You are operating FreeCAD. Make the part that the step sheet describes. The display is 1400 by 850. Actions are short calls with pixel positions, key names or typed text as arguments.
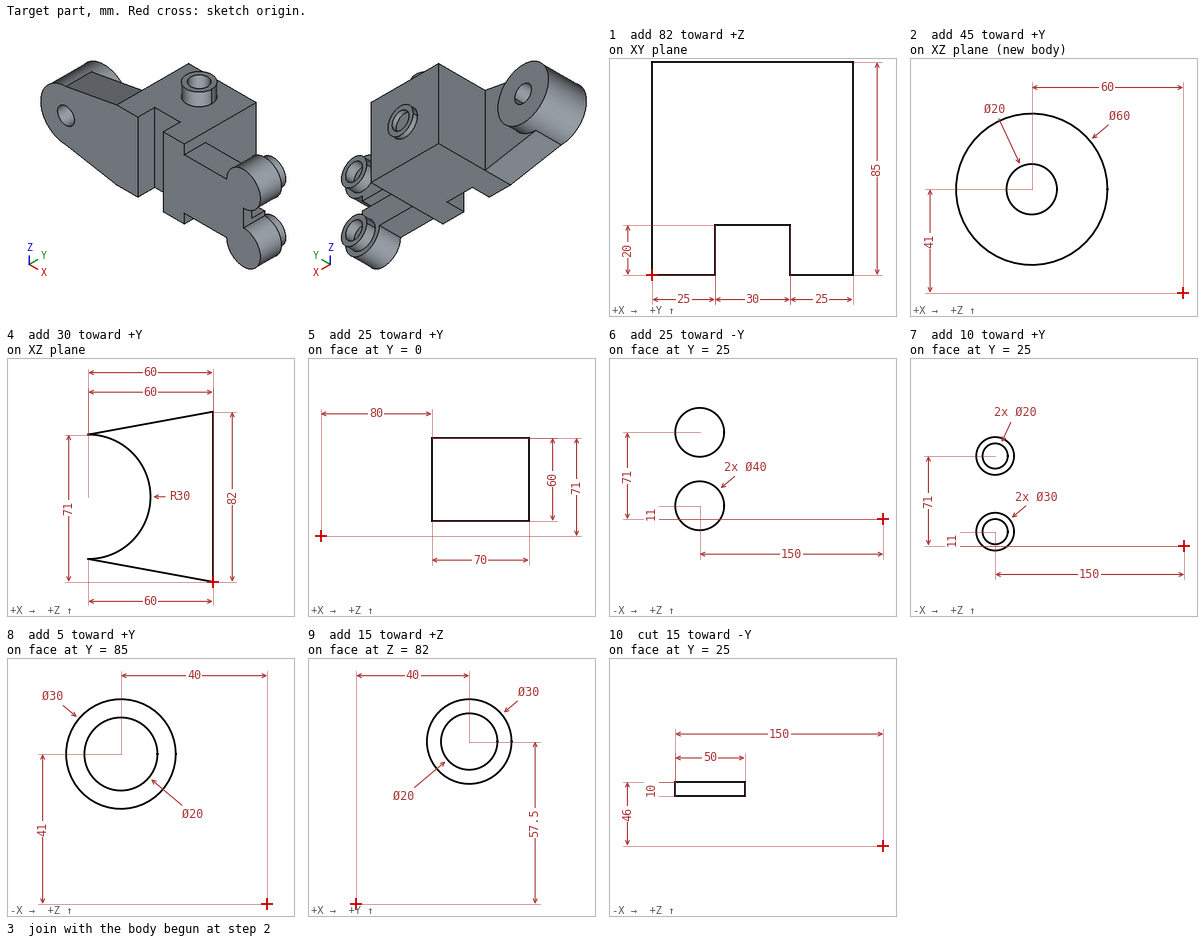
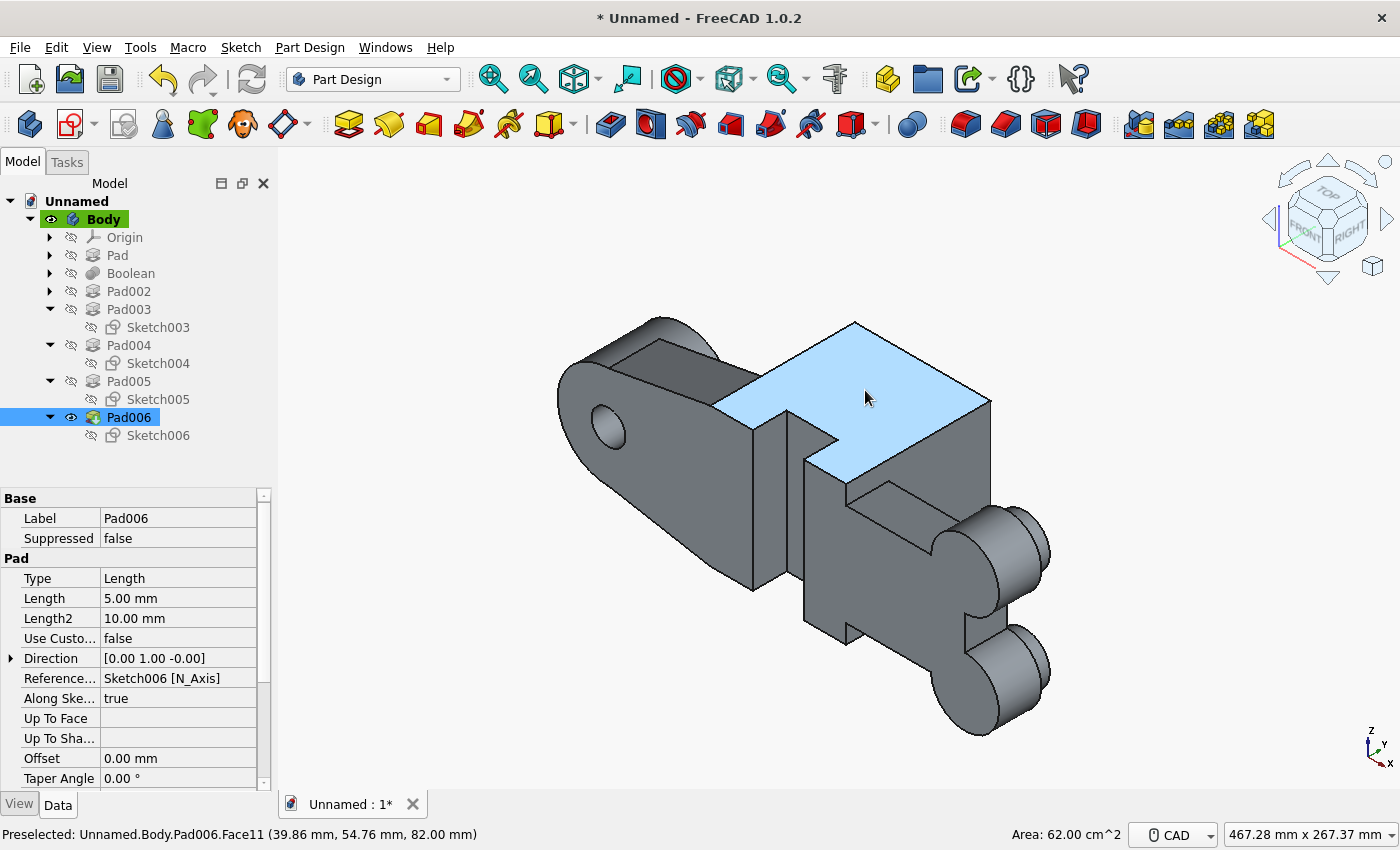
click(70, 124)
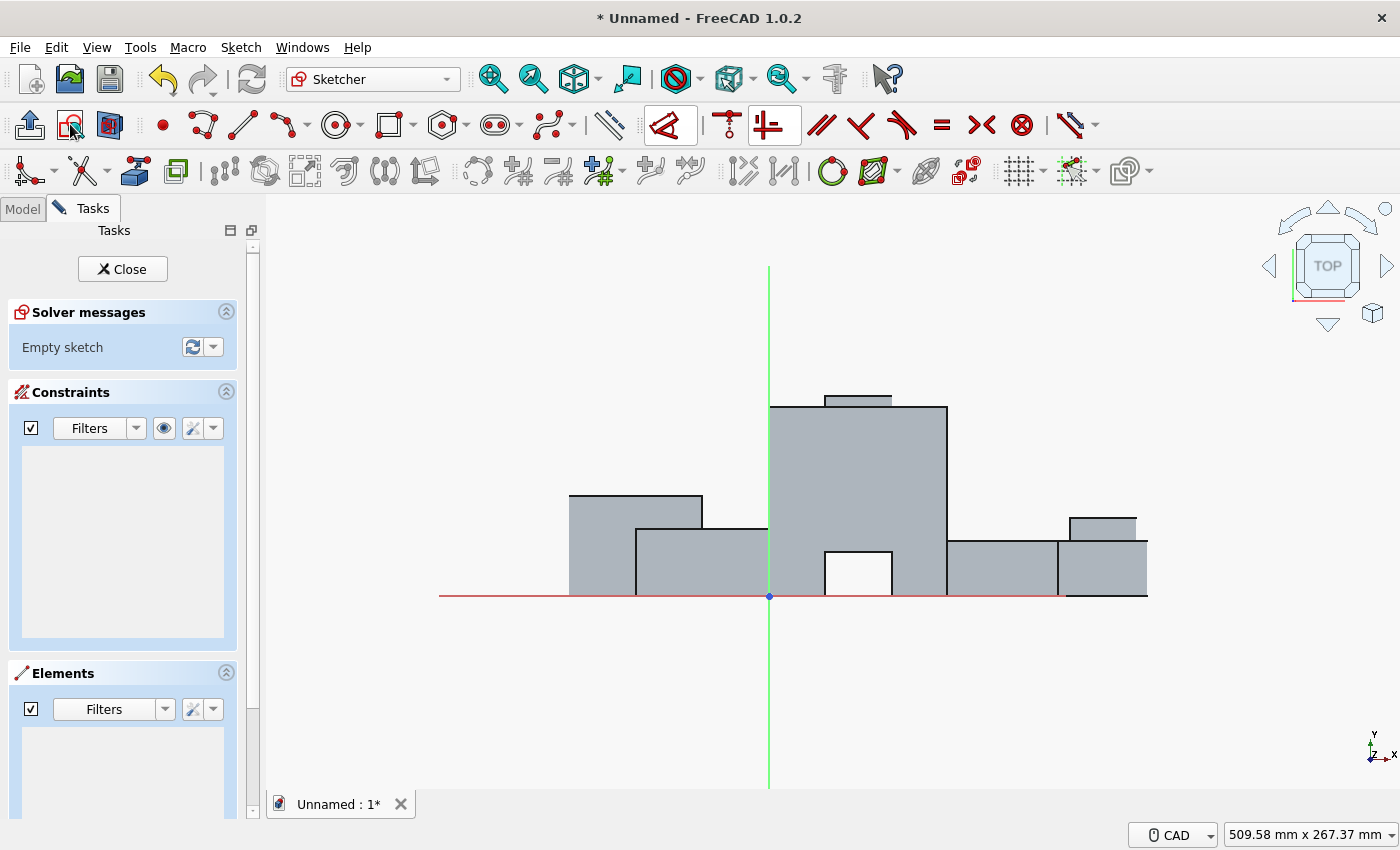
click(110, 126)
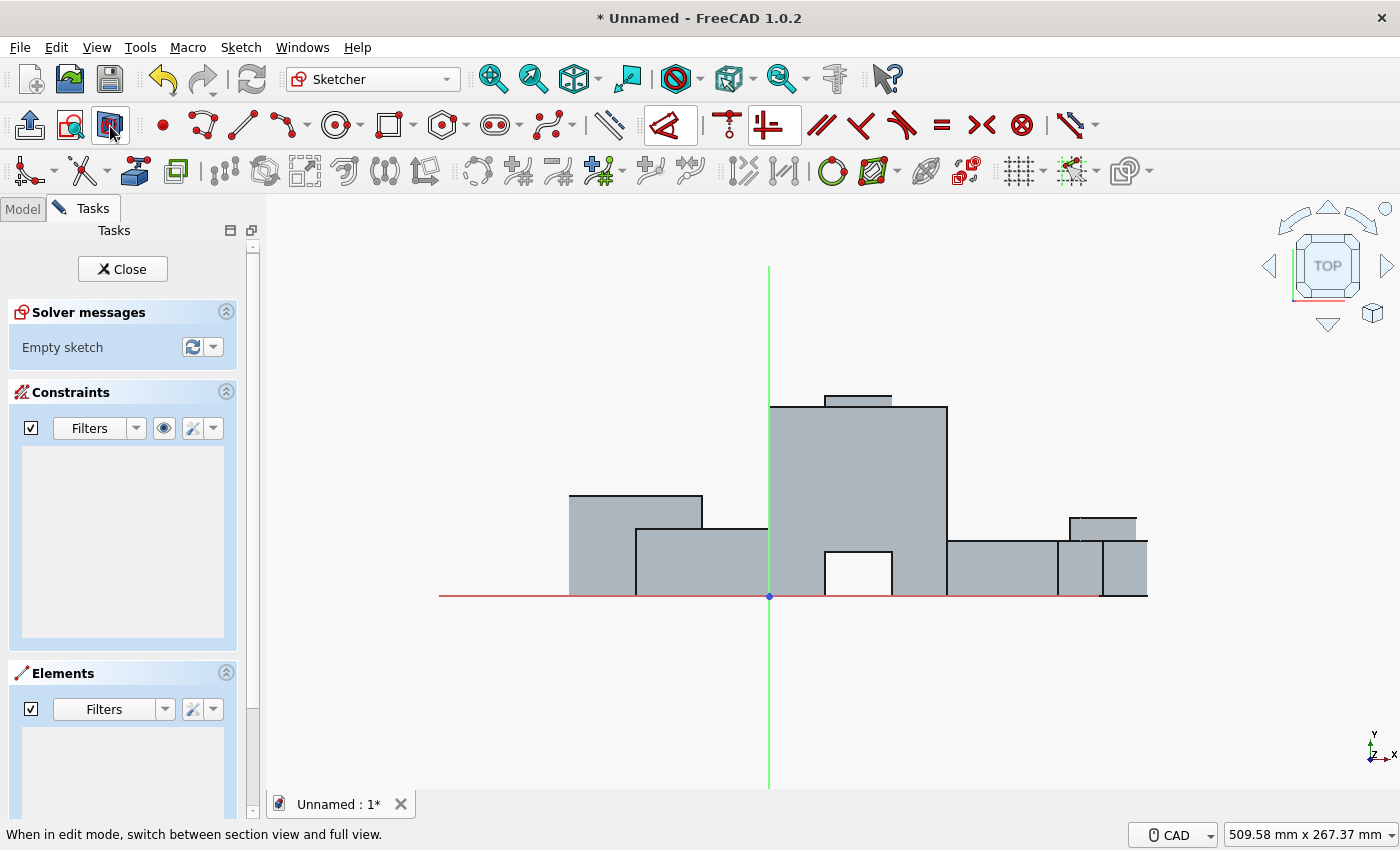
scroll(884, 535, up, 4)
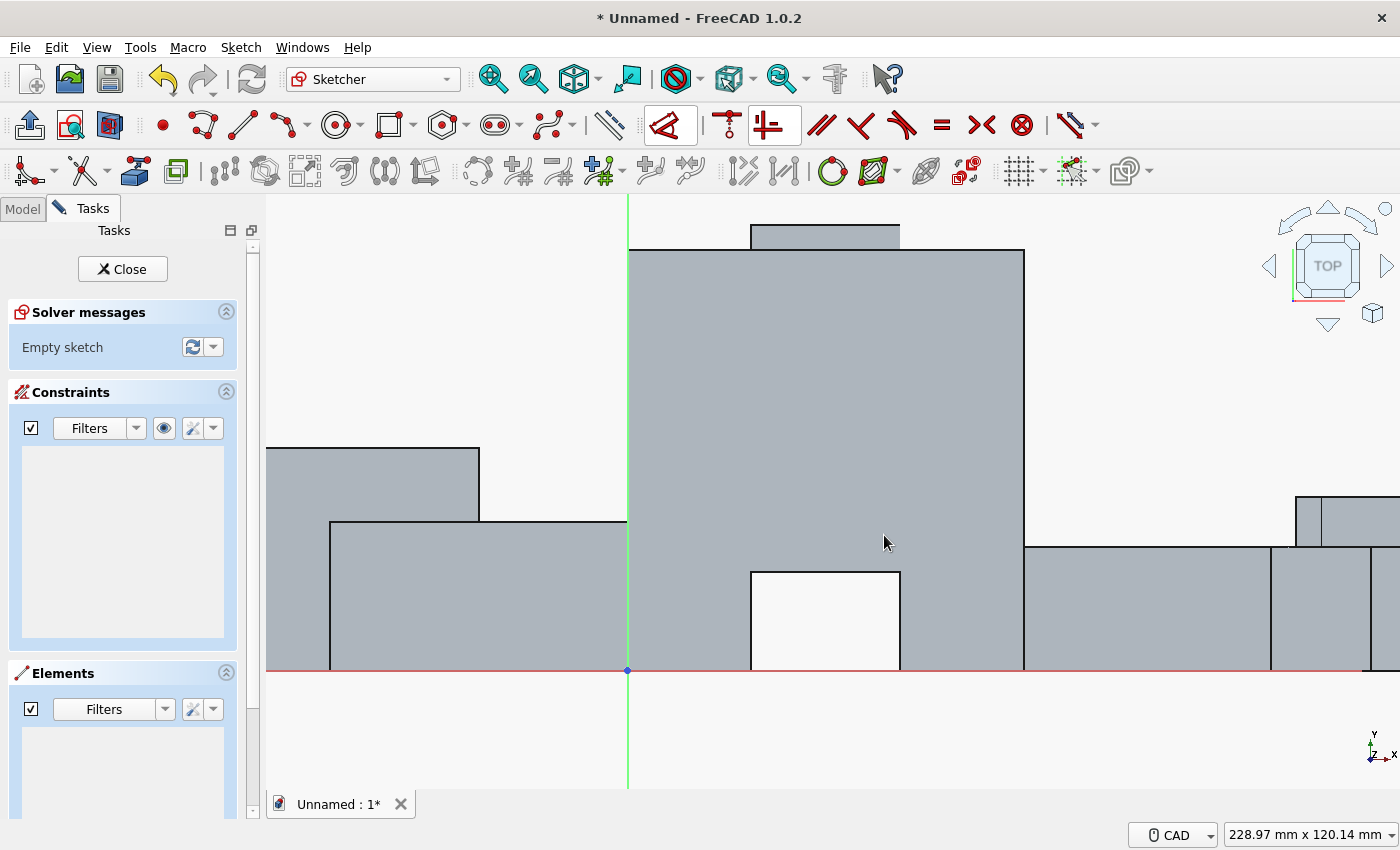
click(336, 126)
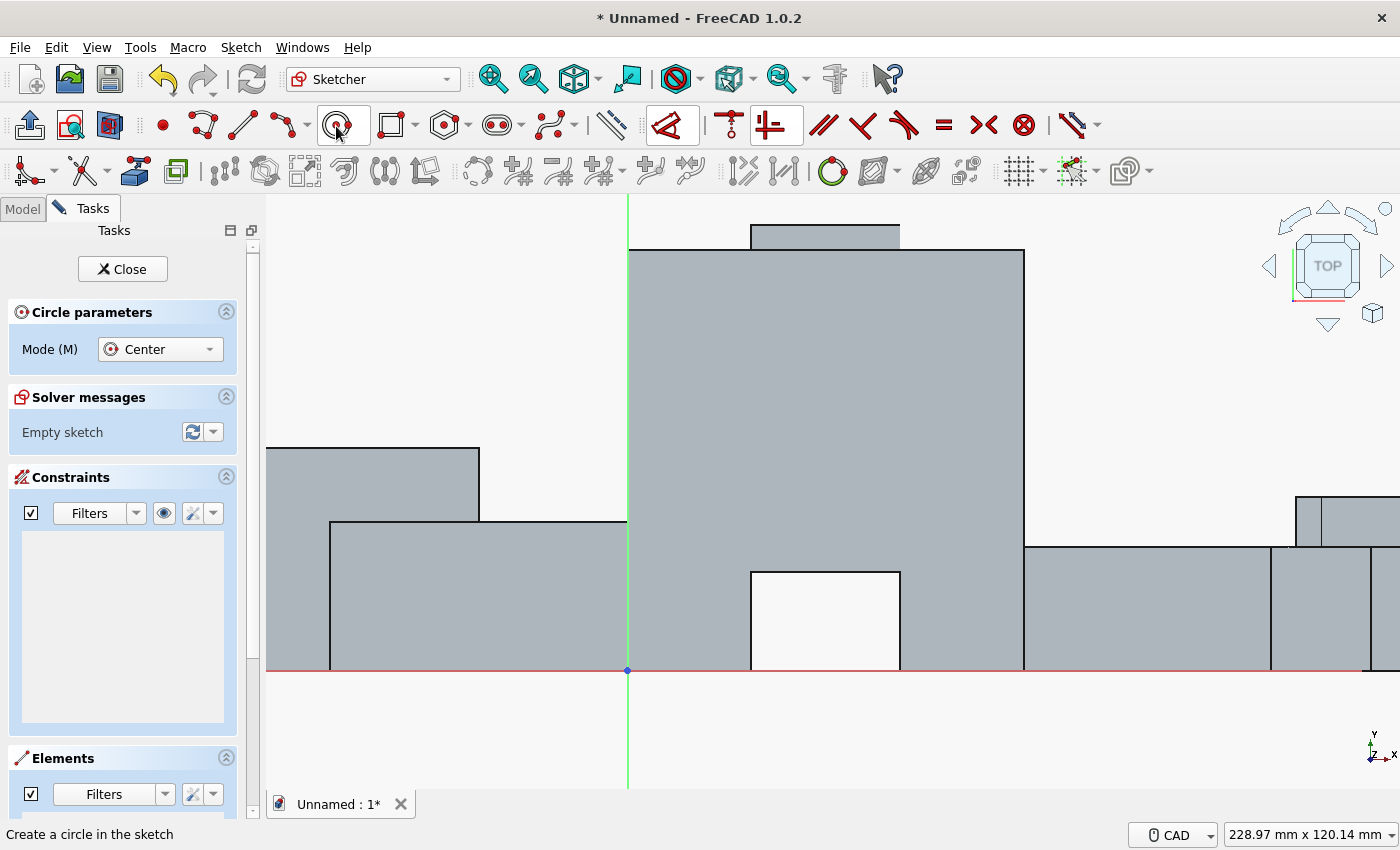
click(826, 386)
click(878, 333)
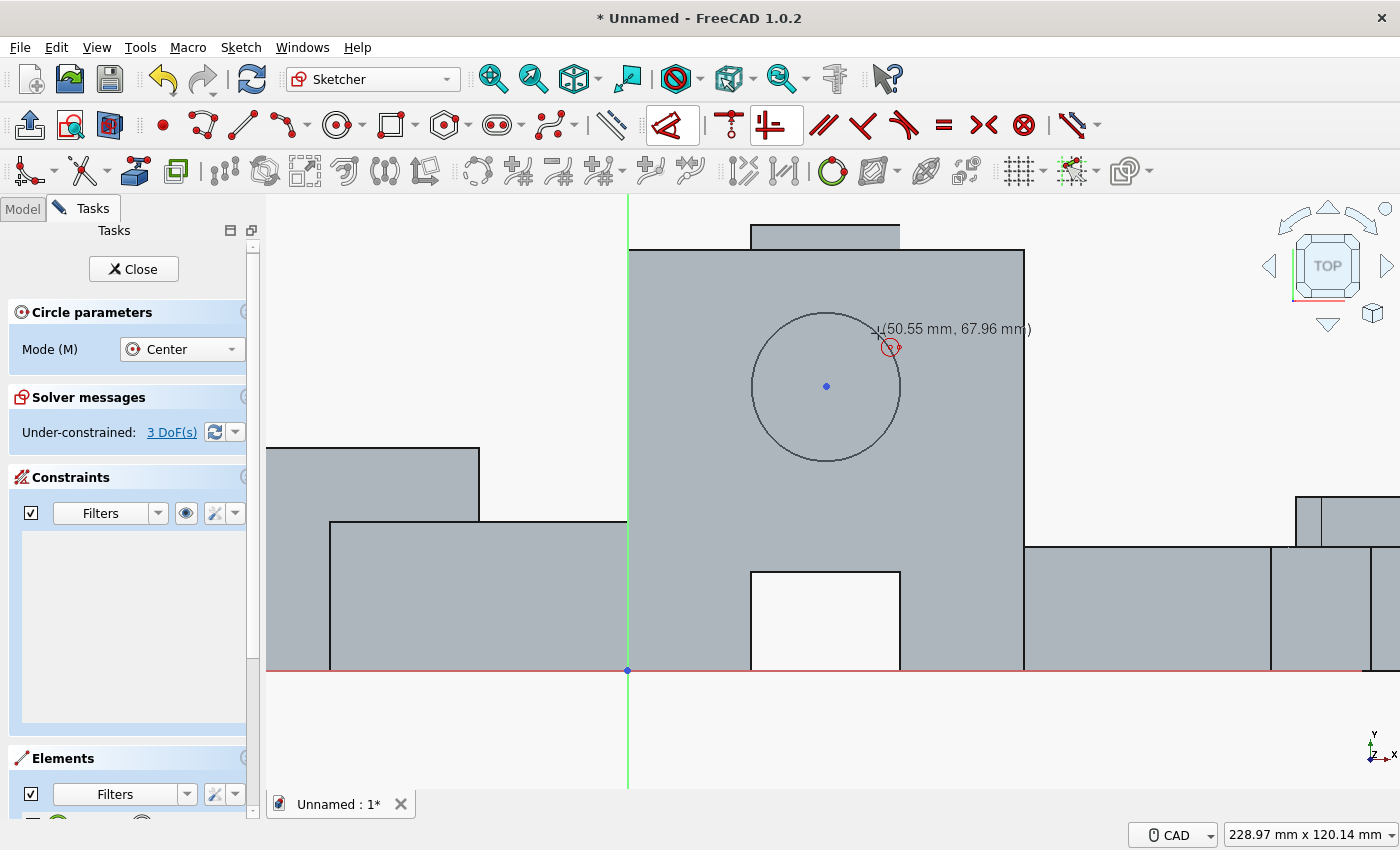
click(826, 387)
click(861, 351)
key(Escape)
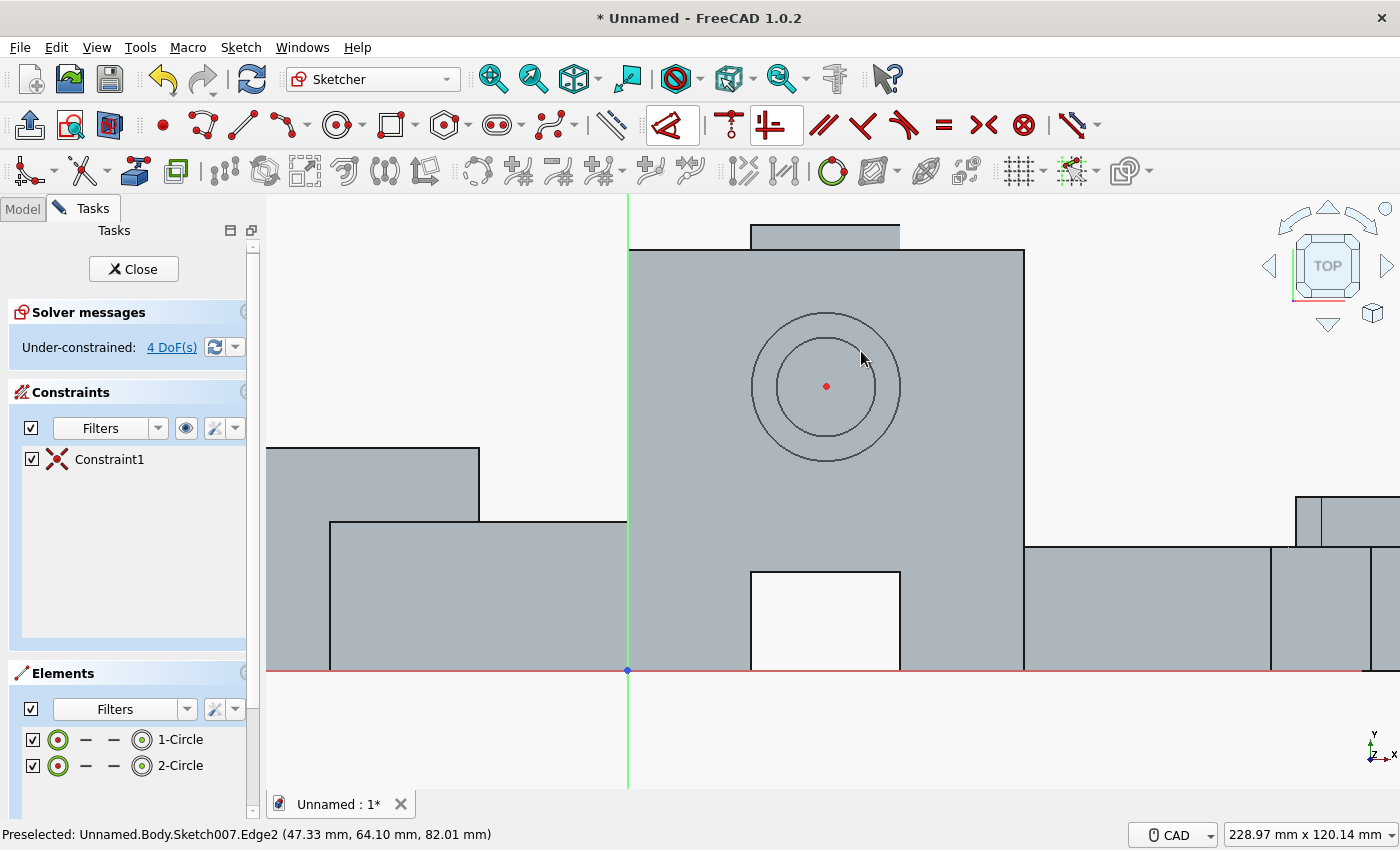
click(878, 334)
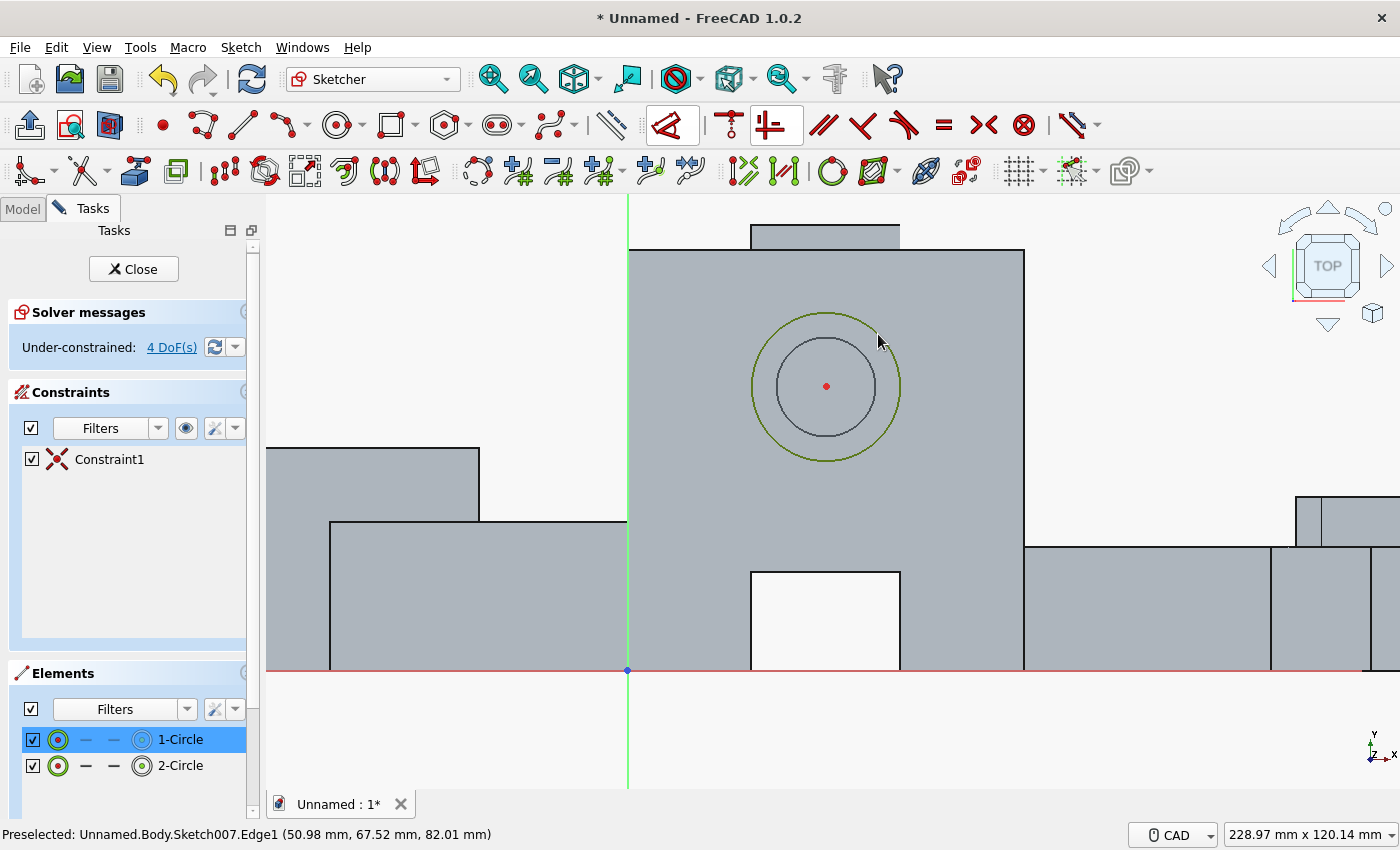
key(k)
key(o)